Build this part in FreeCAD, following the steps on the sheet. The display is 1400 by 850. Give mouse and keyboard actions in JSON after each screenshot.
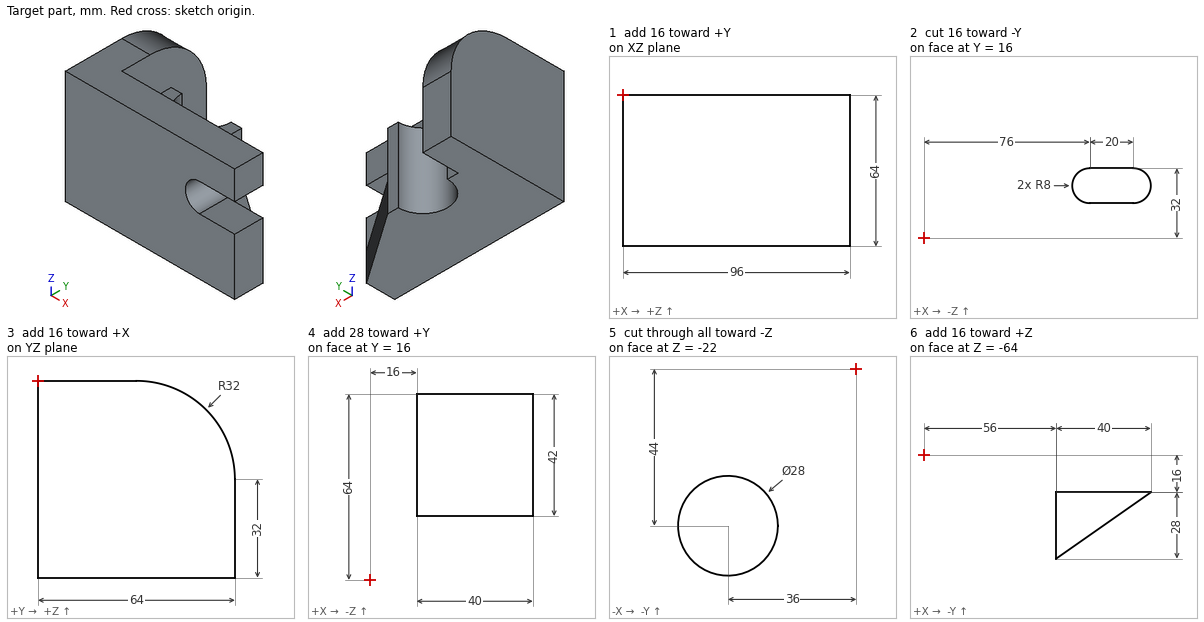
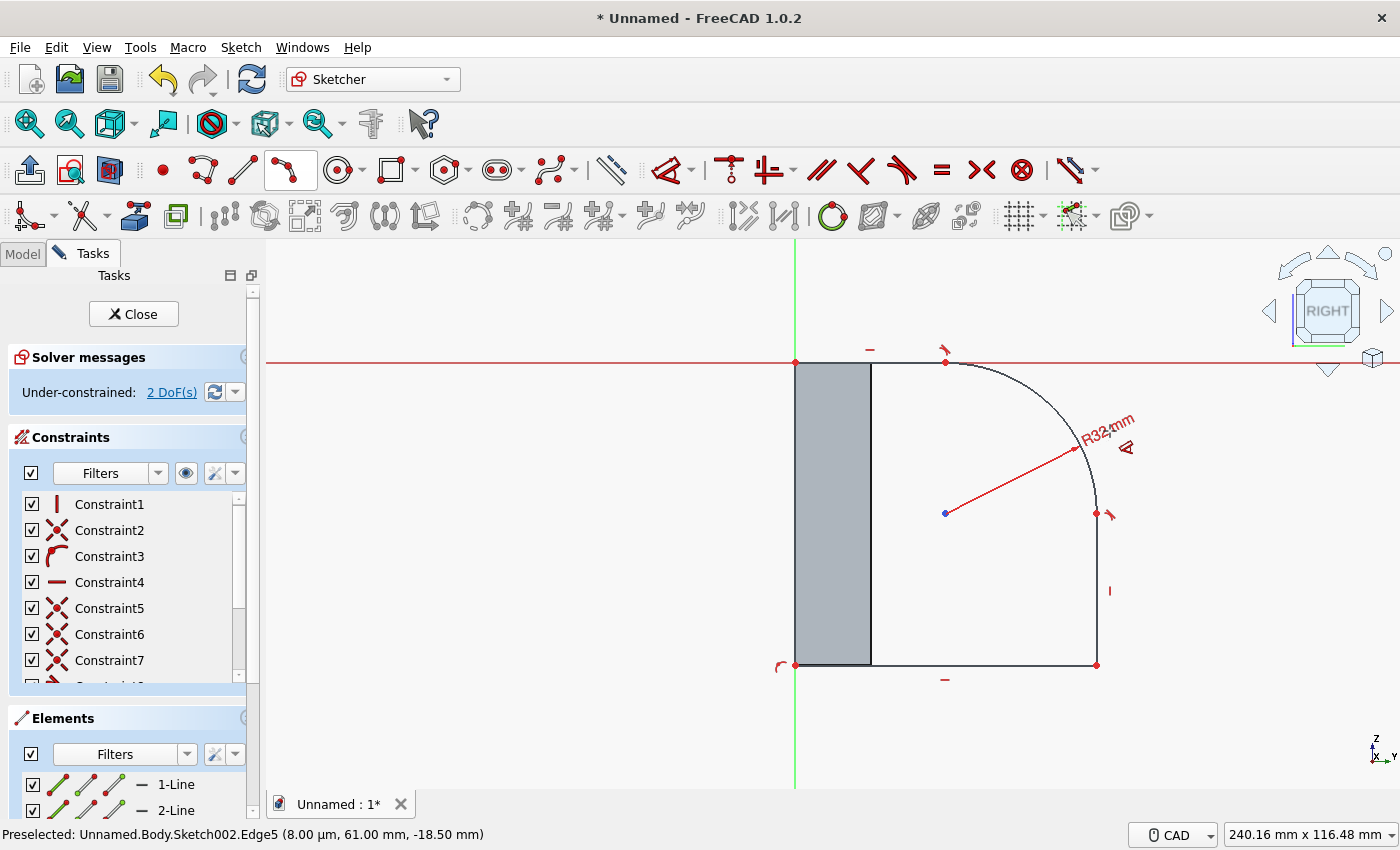
{"action": "left_click", "coordinate": [1097, 560]}
{"action": "left_click", "coordinate": [1131, 590]}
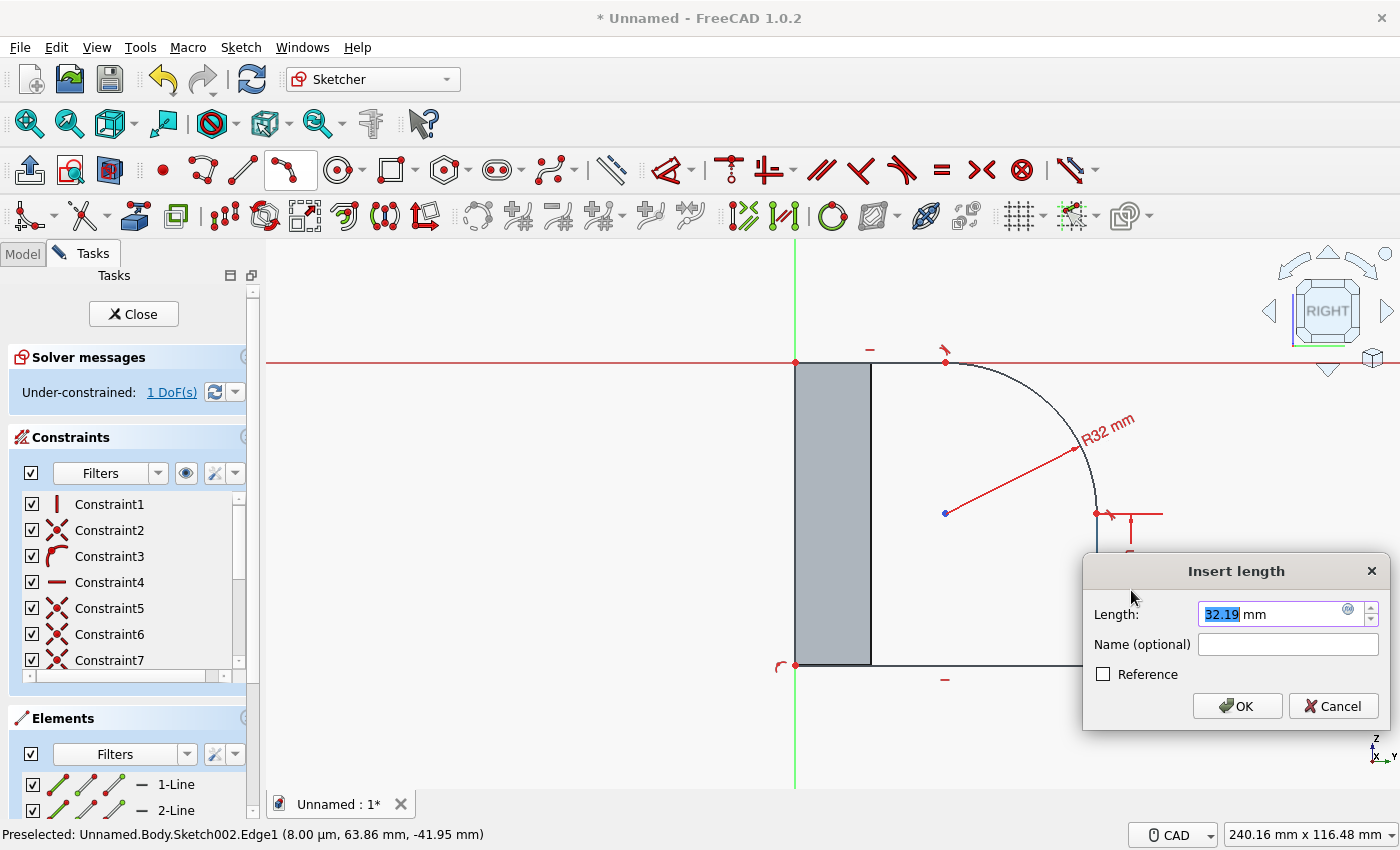
{"action": "type", "text": "32"}
{"action": "key", "text": "Return"}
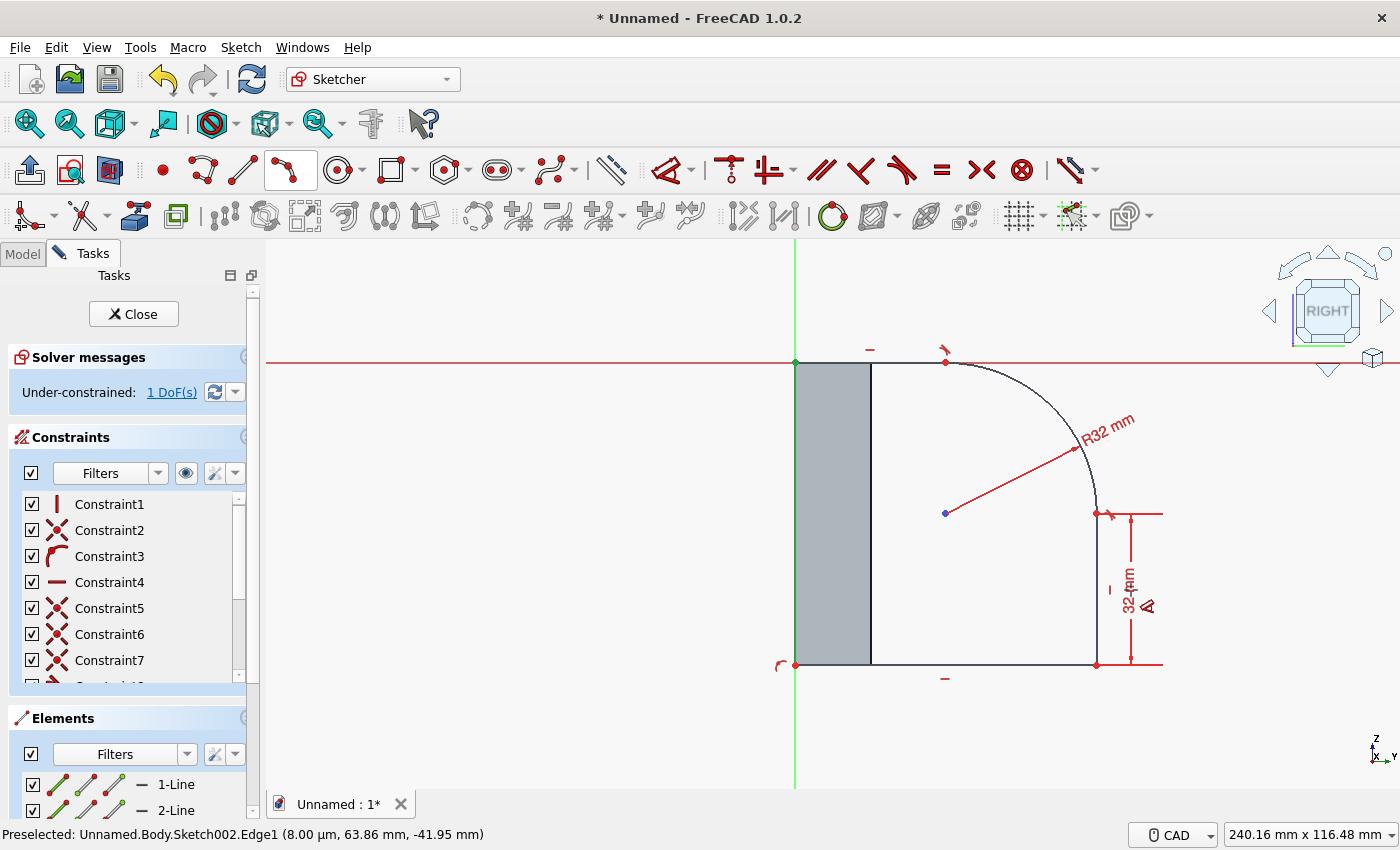
{"action": "left_click", "coordinate": [1006, 665]}
{"action": "left_click", "coordinate": [946, 699]}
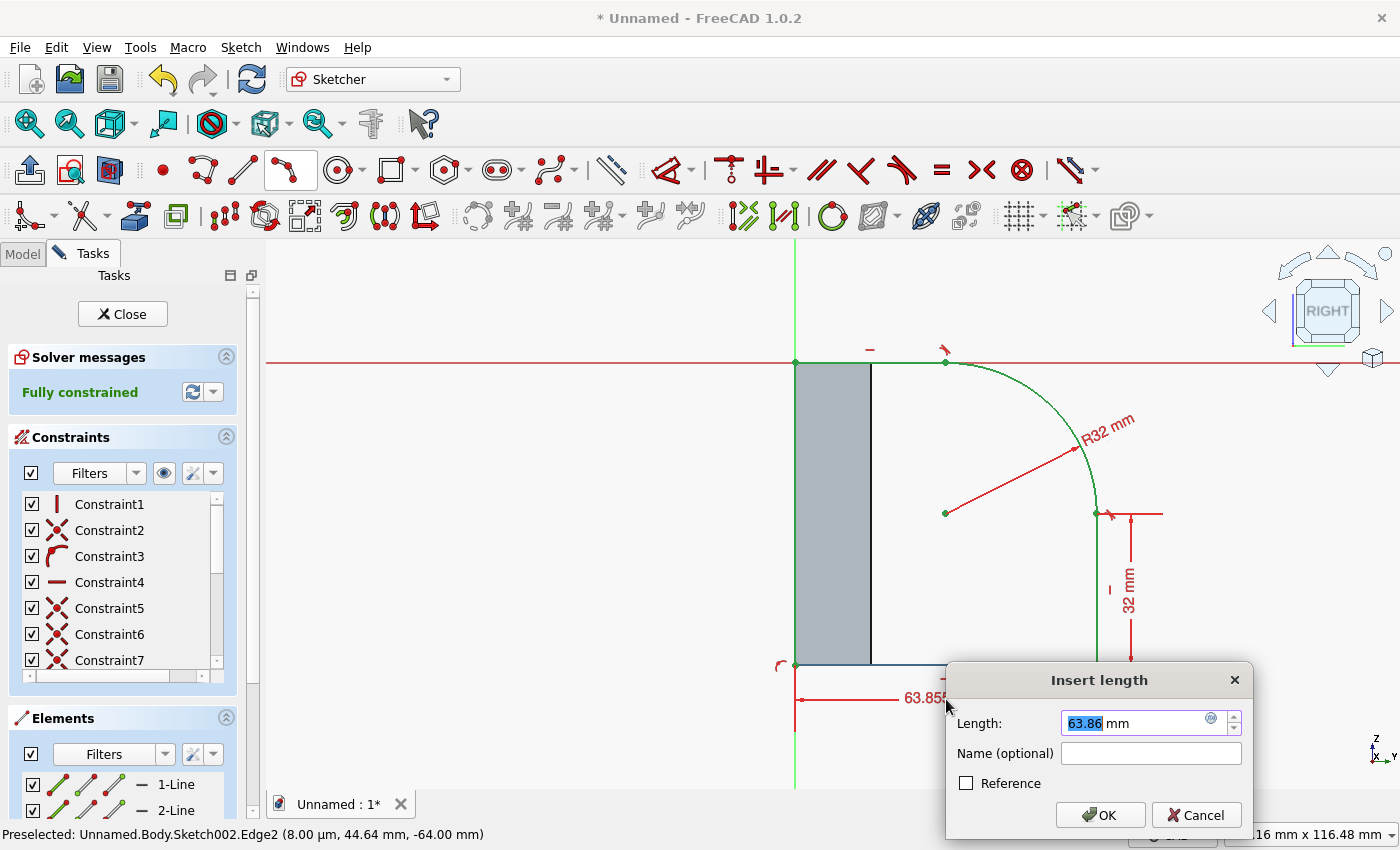
{"action": "type", "text": "64"}
{"action": "key", "text": "Return"}
{"action": "key", "text": "Escape"}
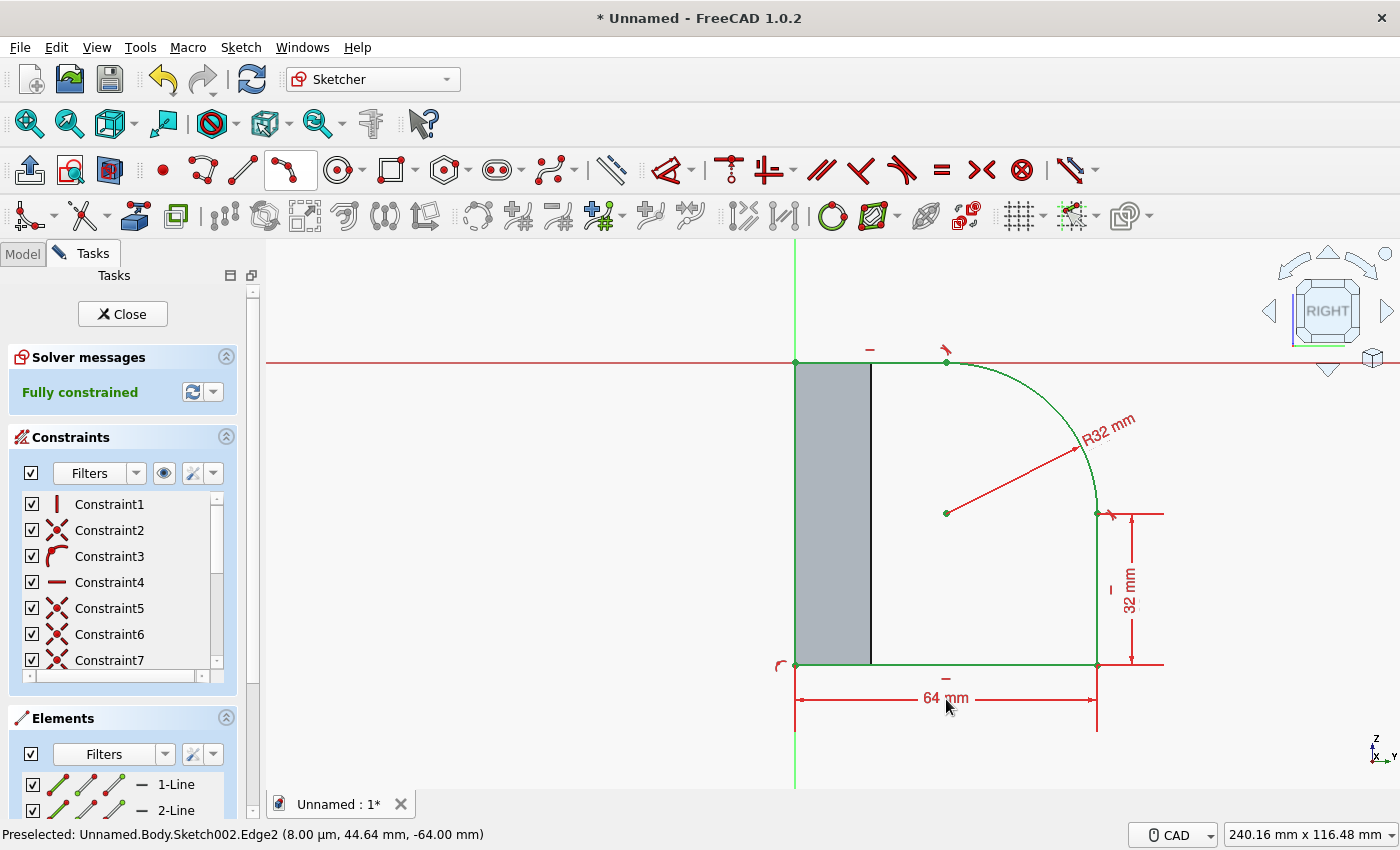
{"action": "left_click", "coordinate": [123, 314]}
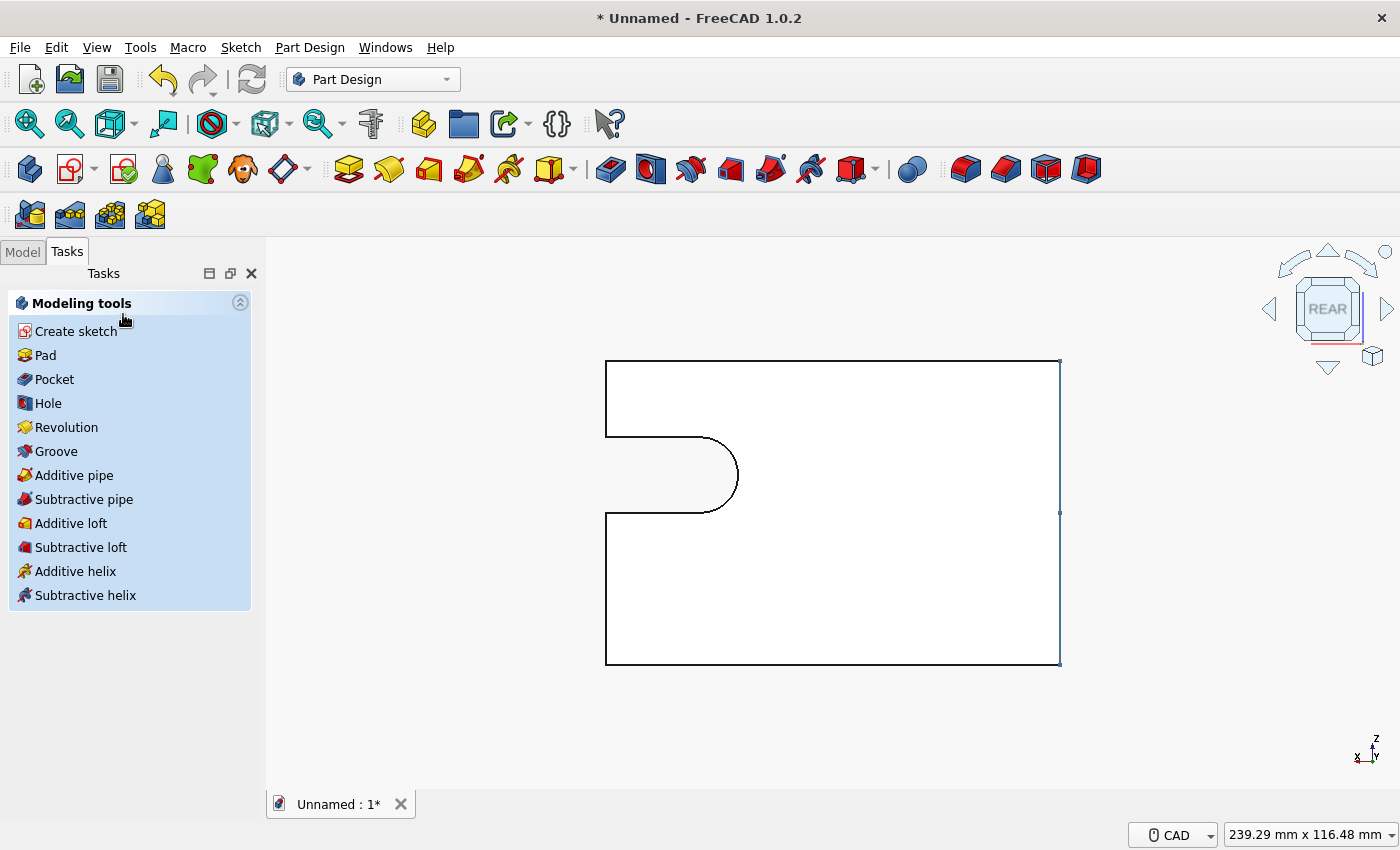
{"action": "left_click", "coordinate": [350, 170]}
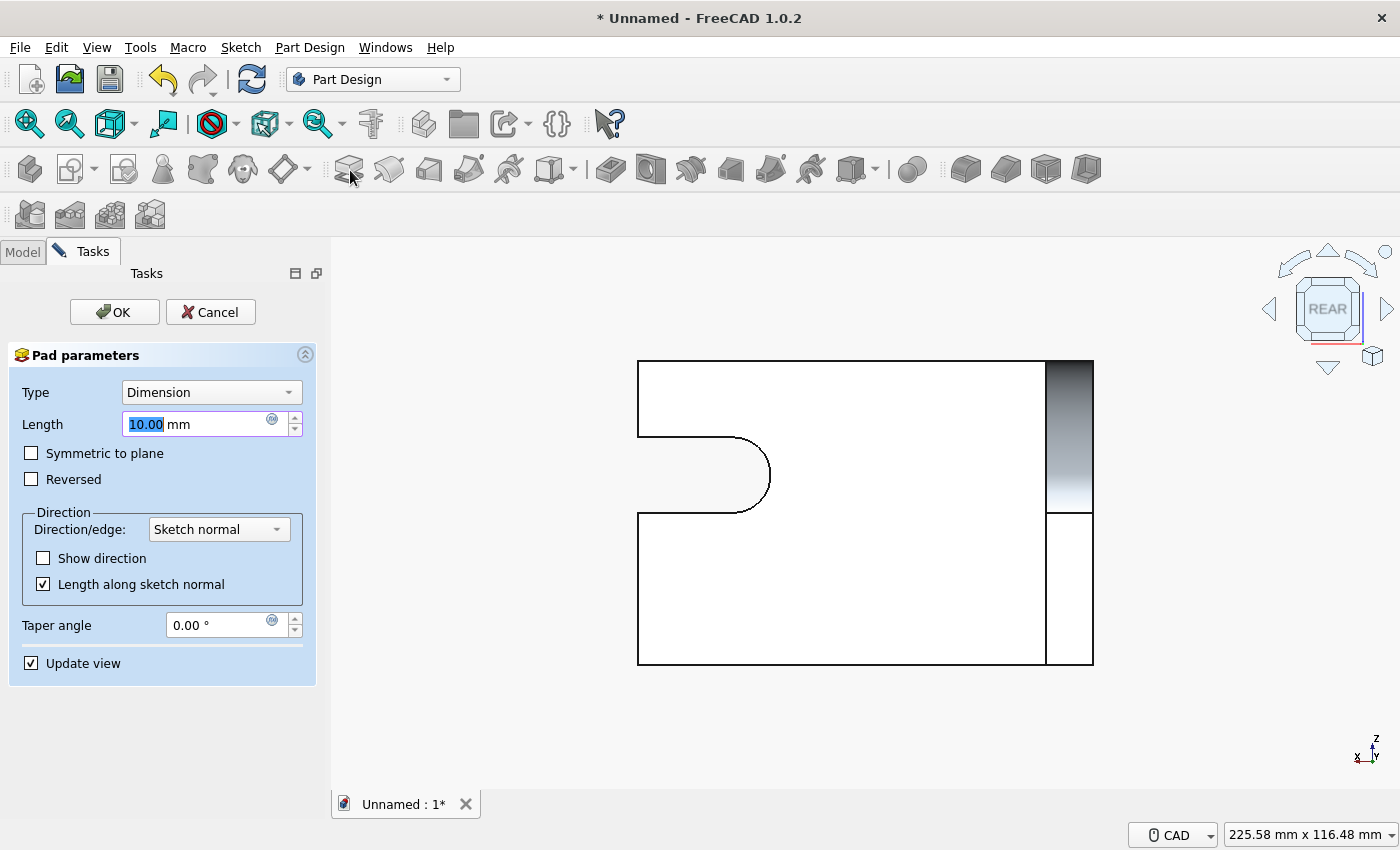
{"action": "type", "text": "16"}
{"action": "key", "text": "Tab"}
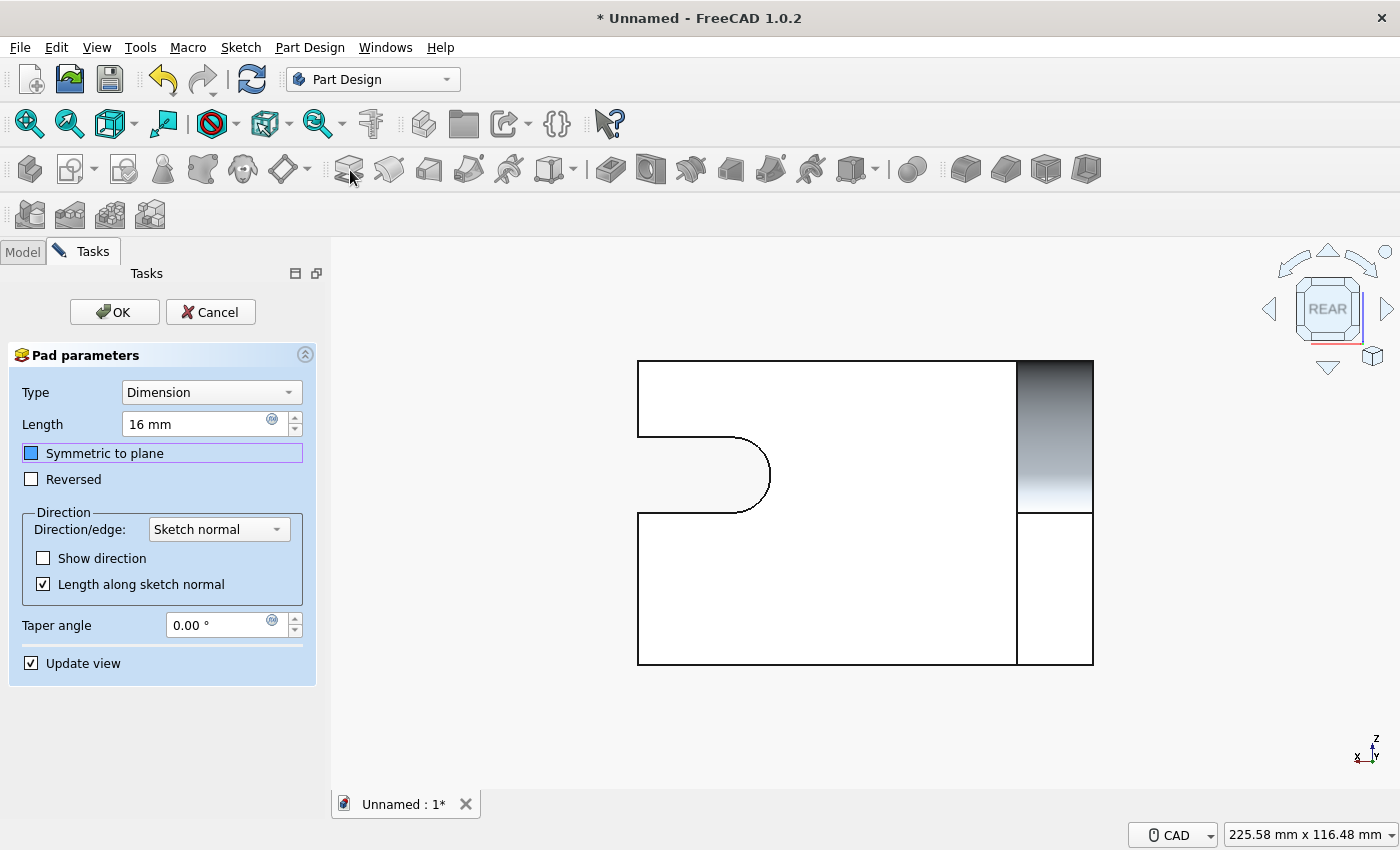
{"action": "left_click", "coordinate": [115, 312]}